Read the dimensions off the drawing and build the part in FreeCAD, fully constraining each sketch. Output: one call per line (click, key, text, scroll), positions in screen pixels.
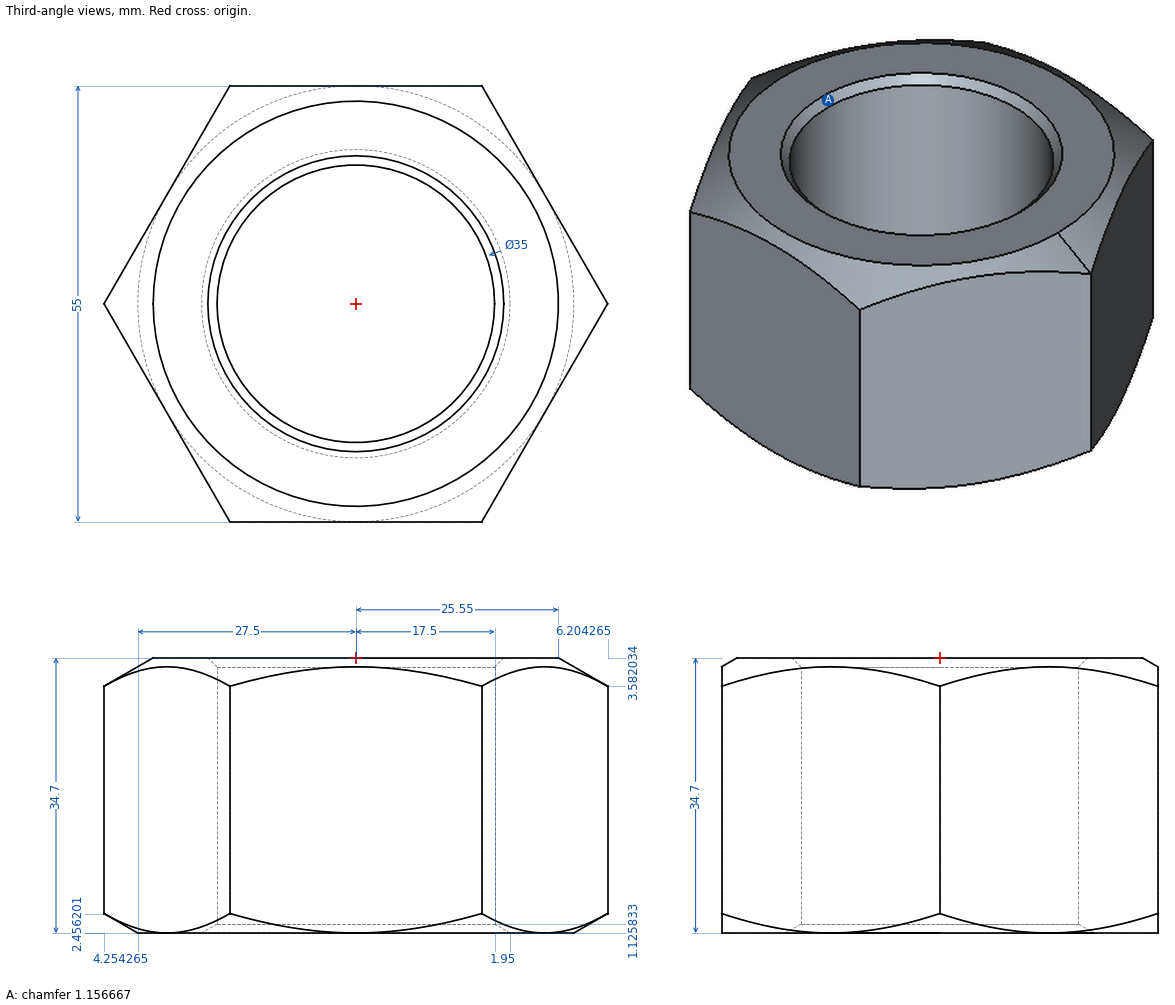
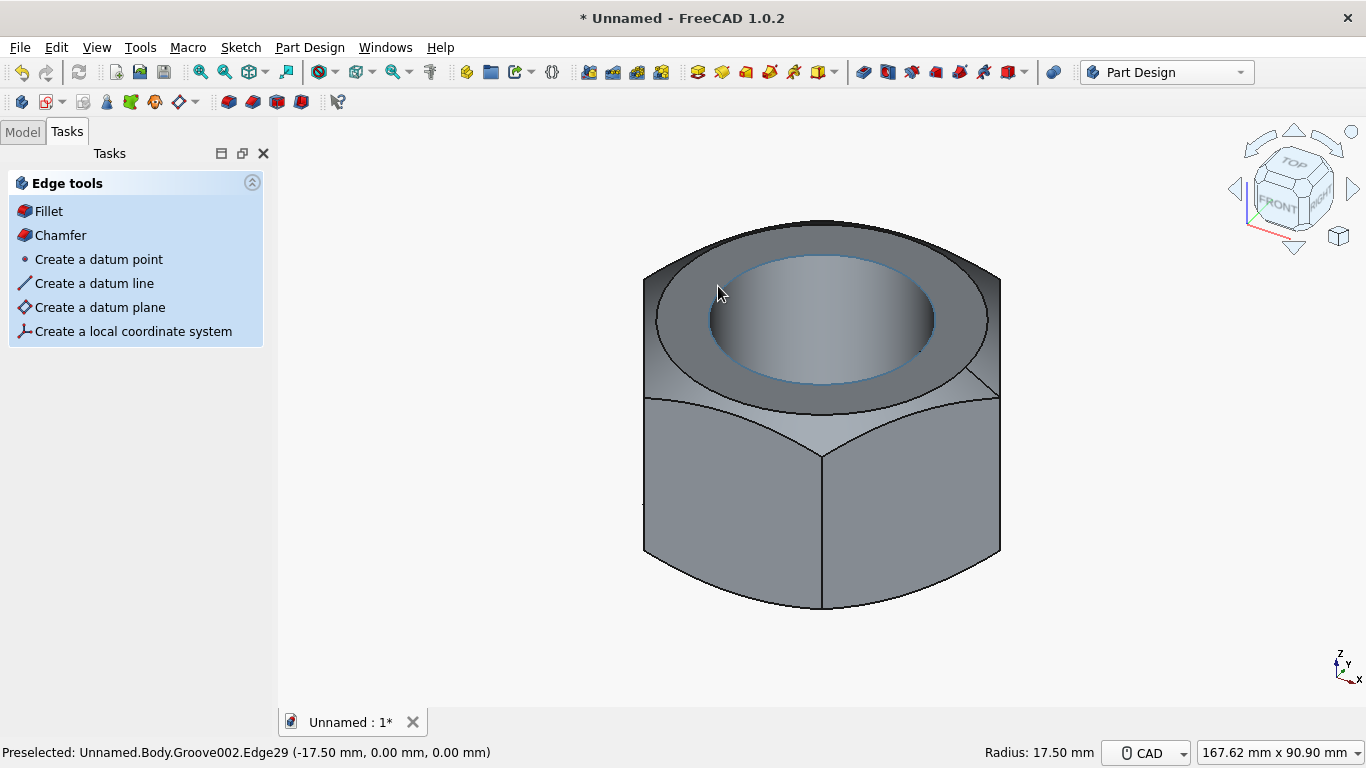
click(254, 102)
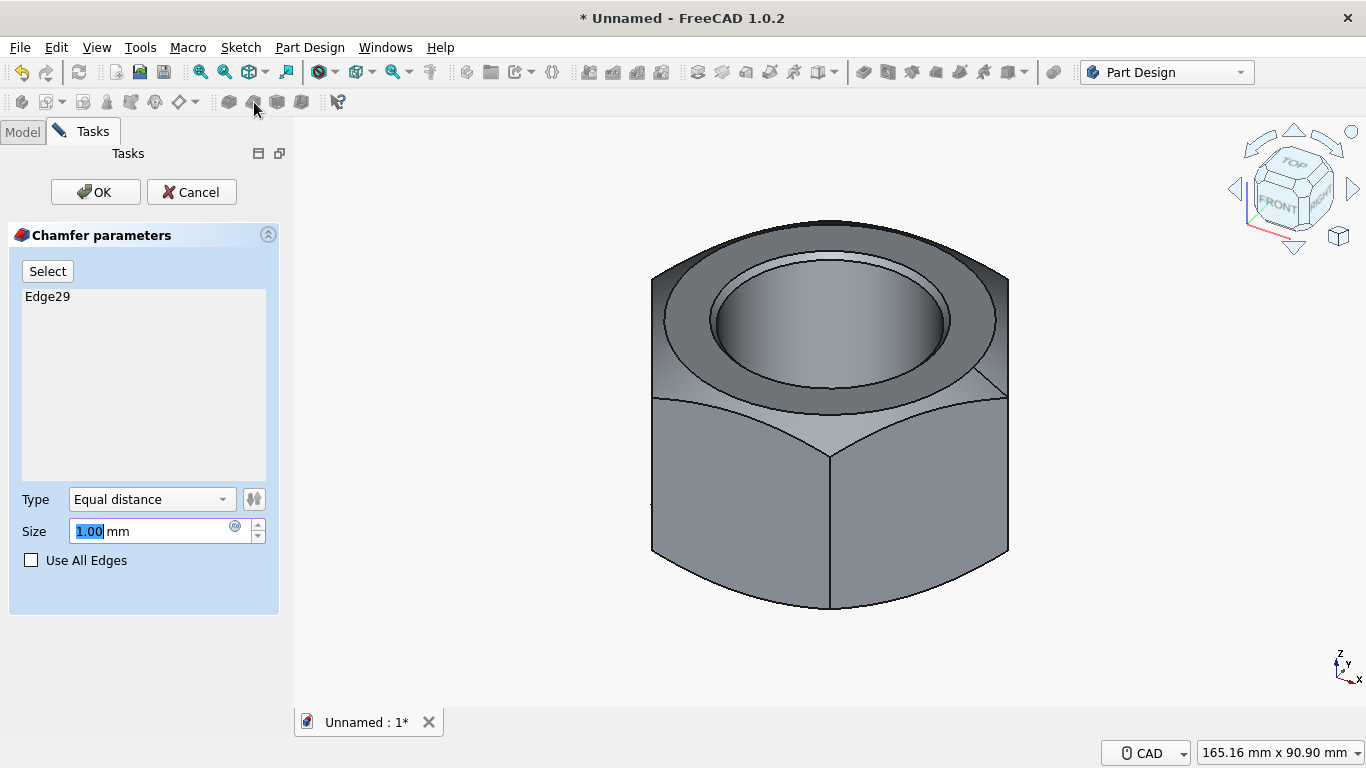
text(1.156667)
key(Tab)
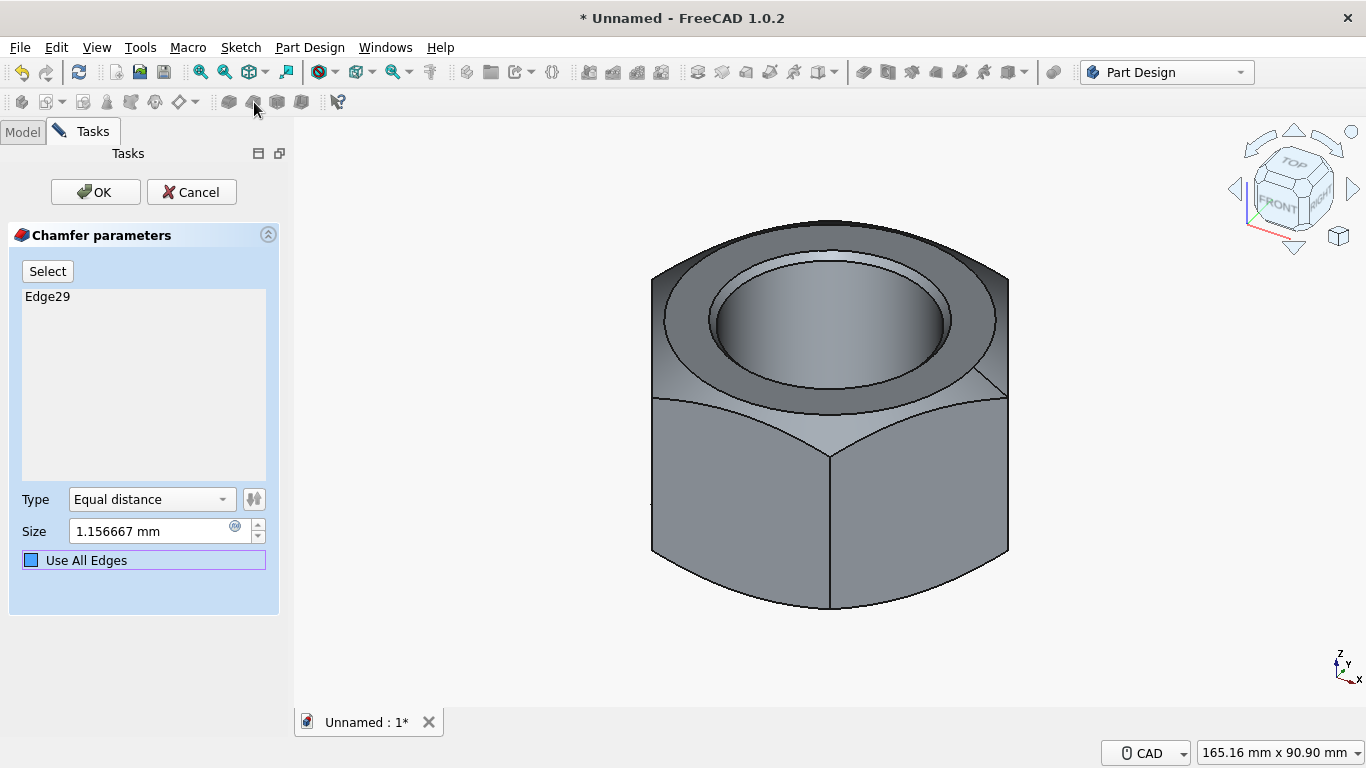
click(96, 192)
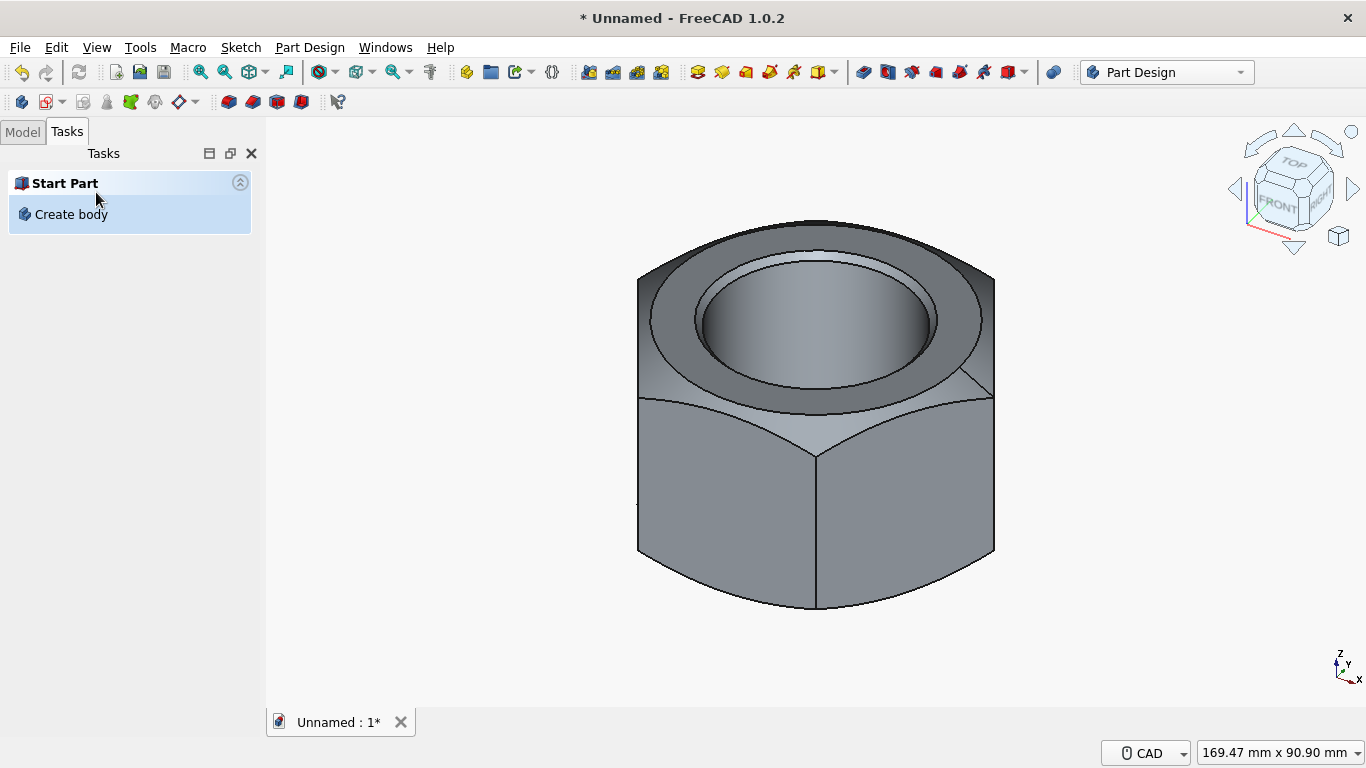
key(0)